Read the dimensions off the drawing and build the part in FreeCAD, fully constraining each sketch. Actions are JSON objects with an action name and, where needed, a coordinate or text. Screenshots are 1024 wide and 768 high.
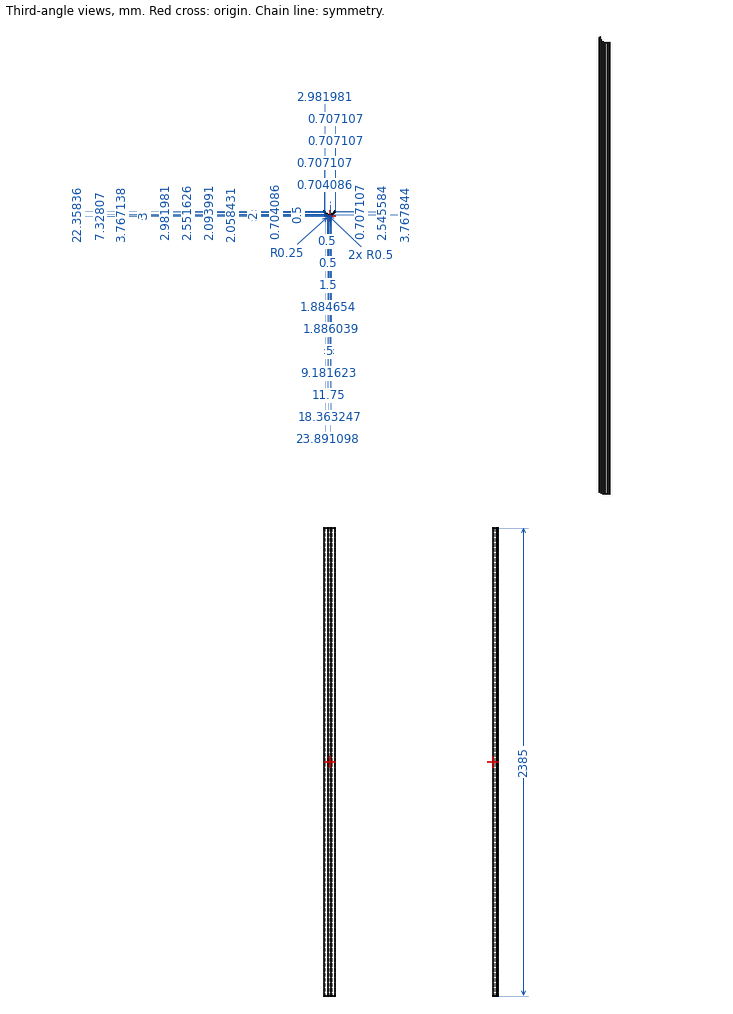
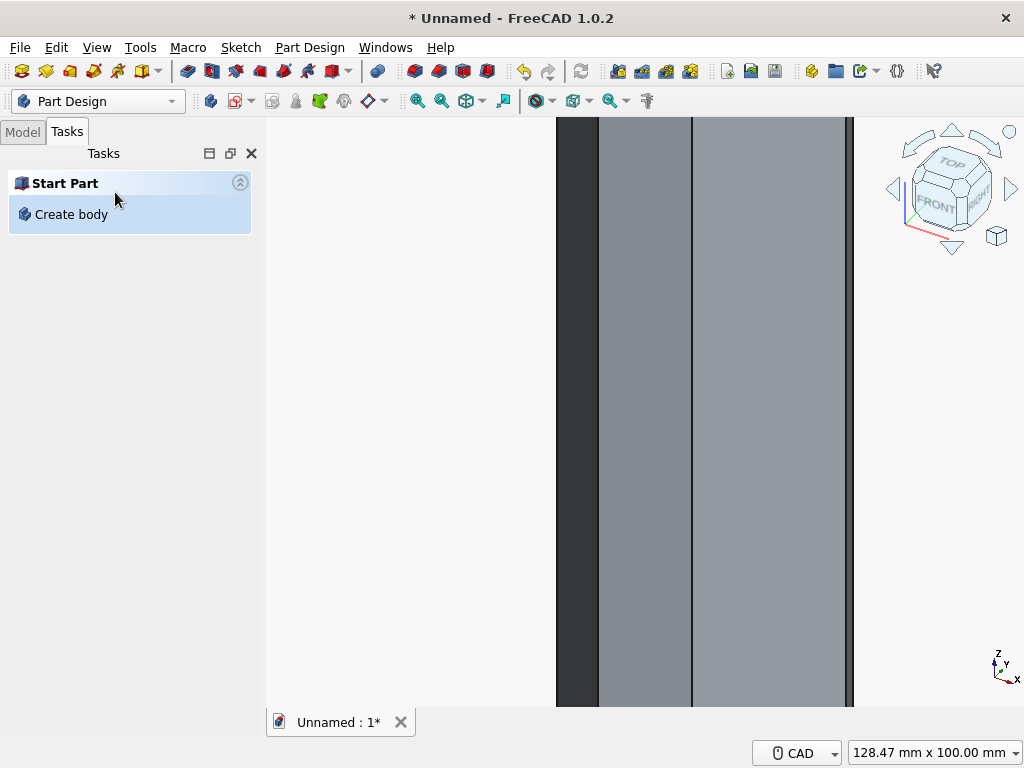
{"action": "key", "text": "0"}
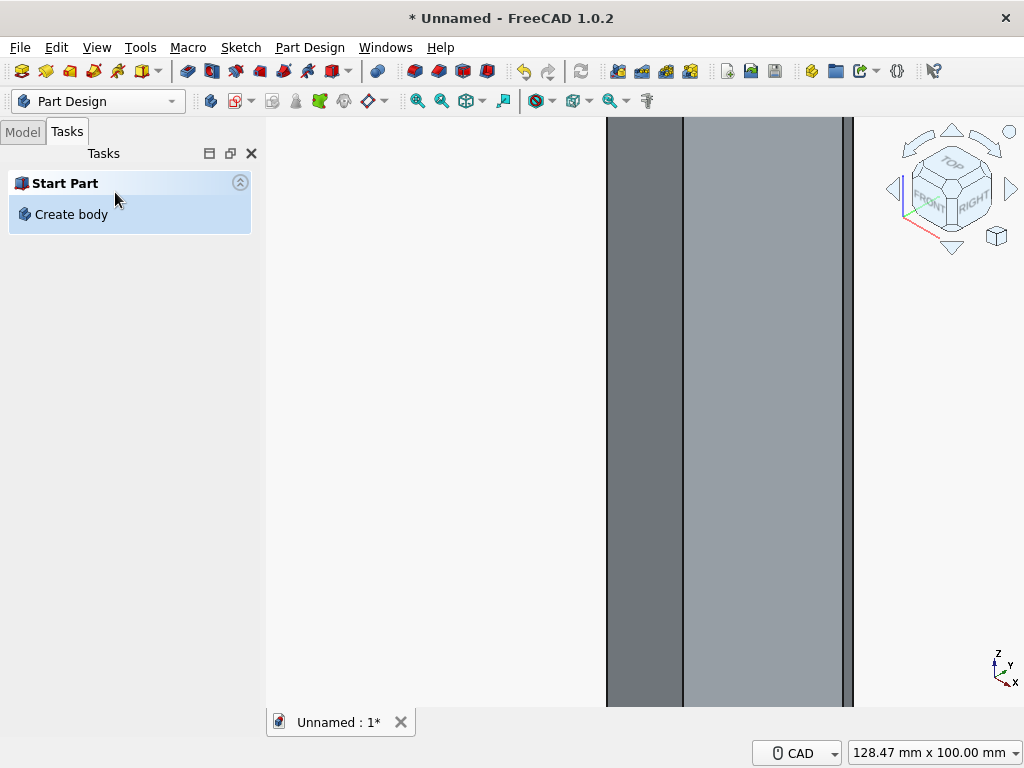
{"action": "key", "text": "v f"}